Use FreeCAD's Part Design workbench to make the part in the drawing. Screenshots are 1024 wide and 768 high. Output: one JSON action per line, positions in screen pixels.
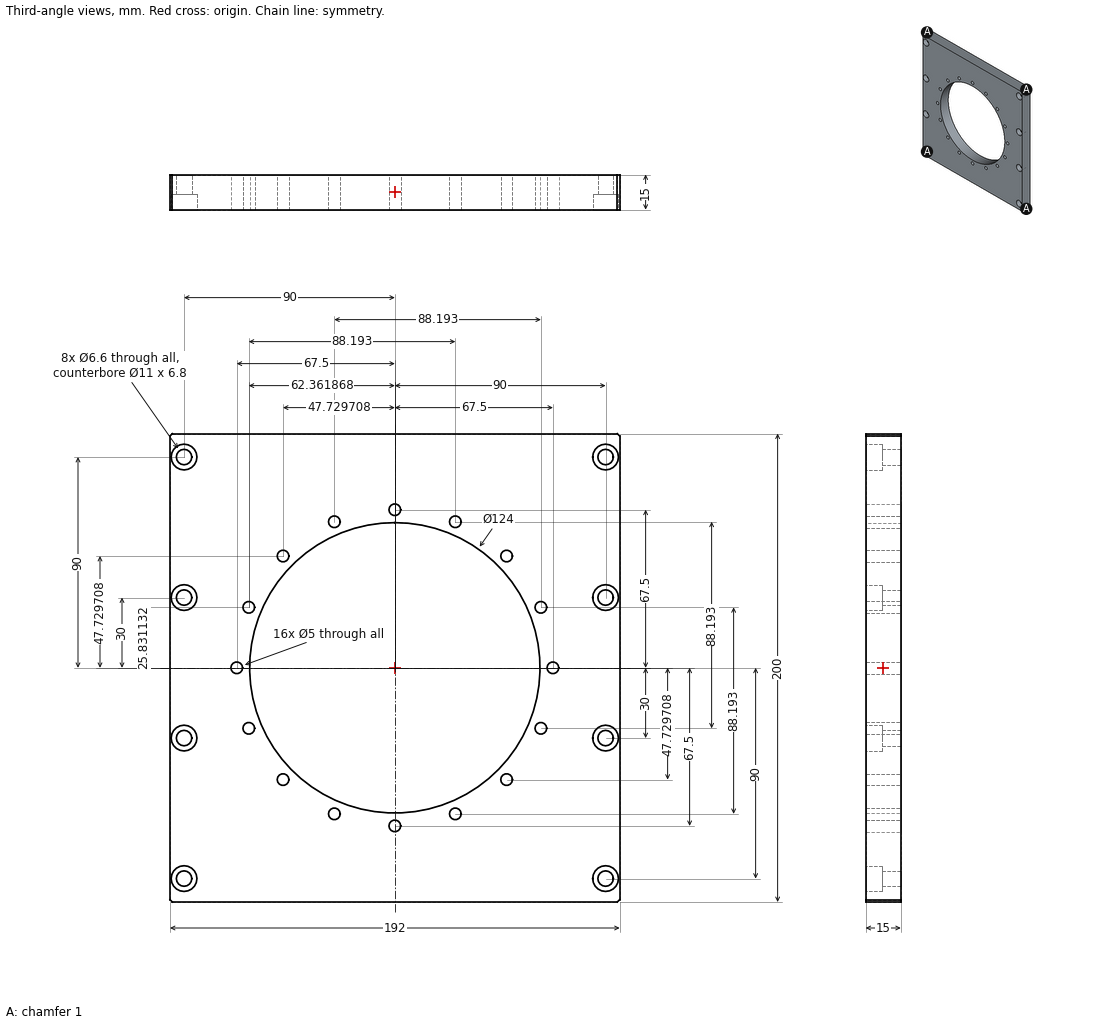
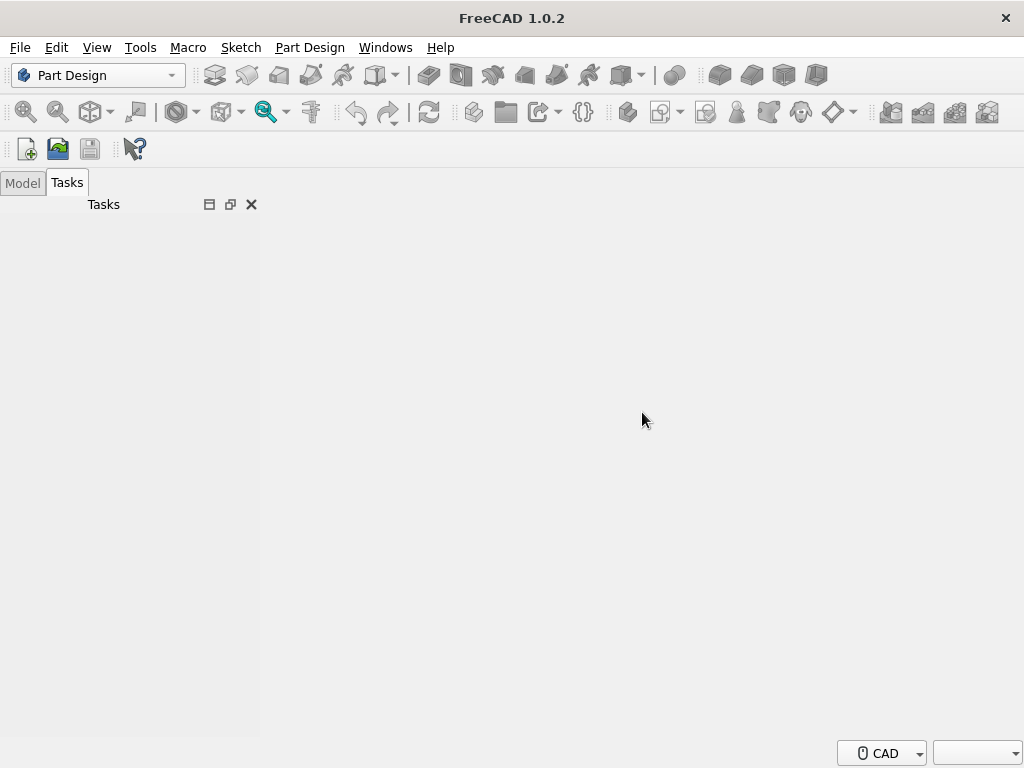
{"action": "left_click", "coordinate": [26, 150]}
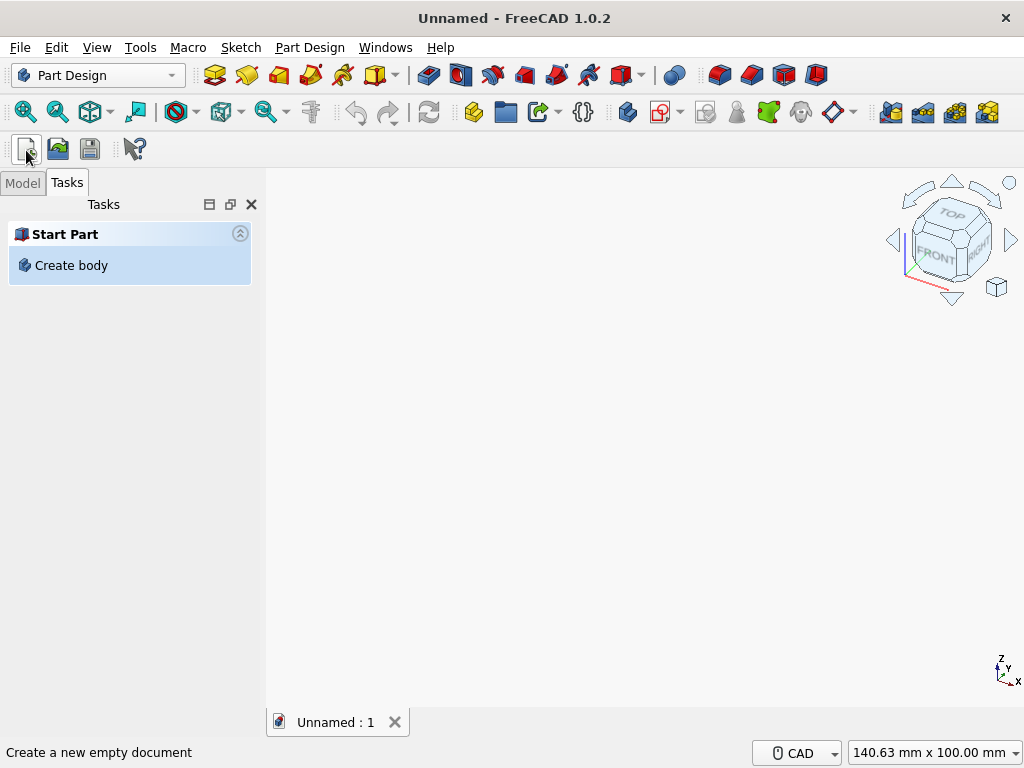
{"action": "left_click", "coordinate": [660, 112]}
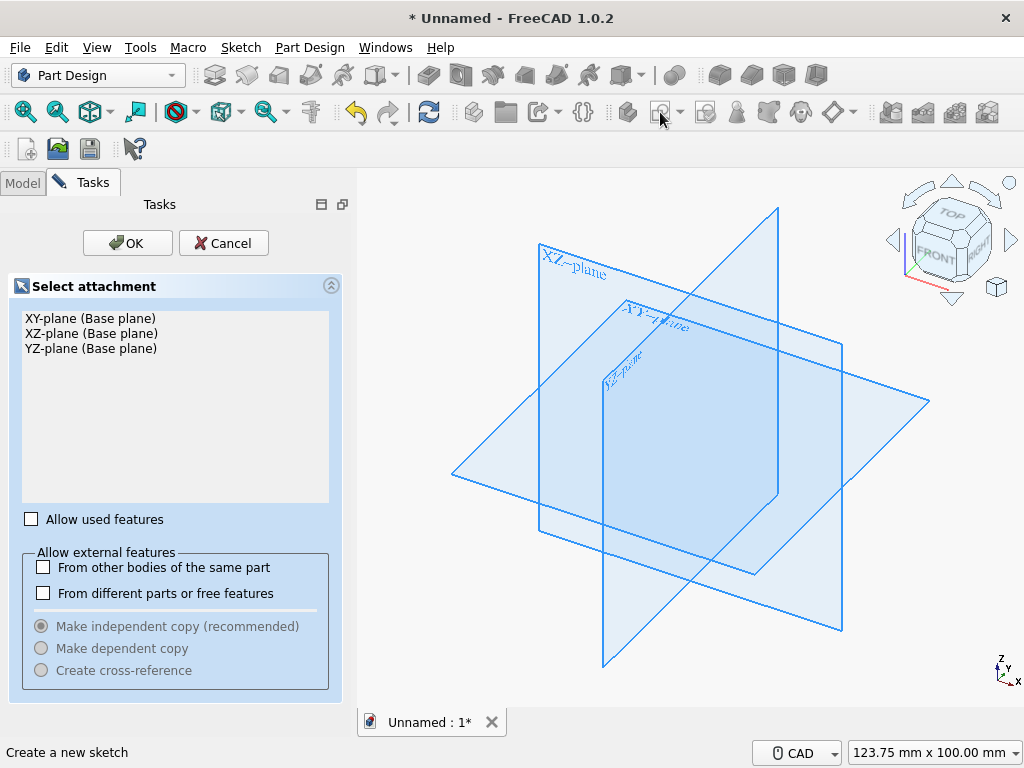
{"action": "left_click", "coordinate": [82, 334]}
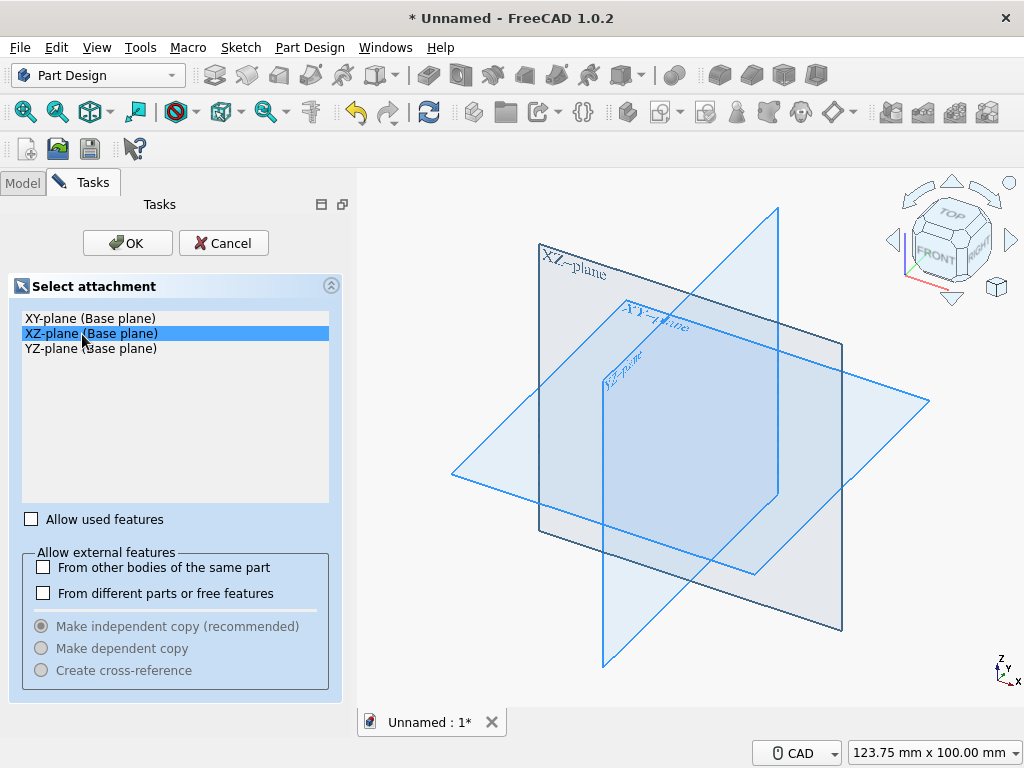
{"action": "left_click", "coordinate": [128, 243]}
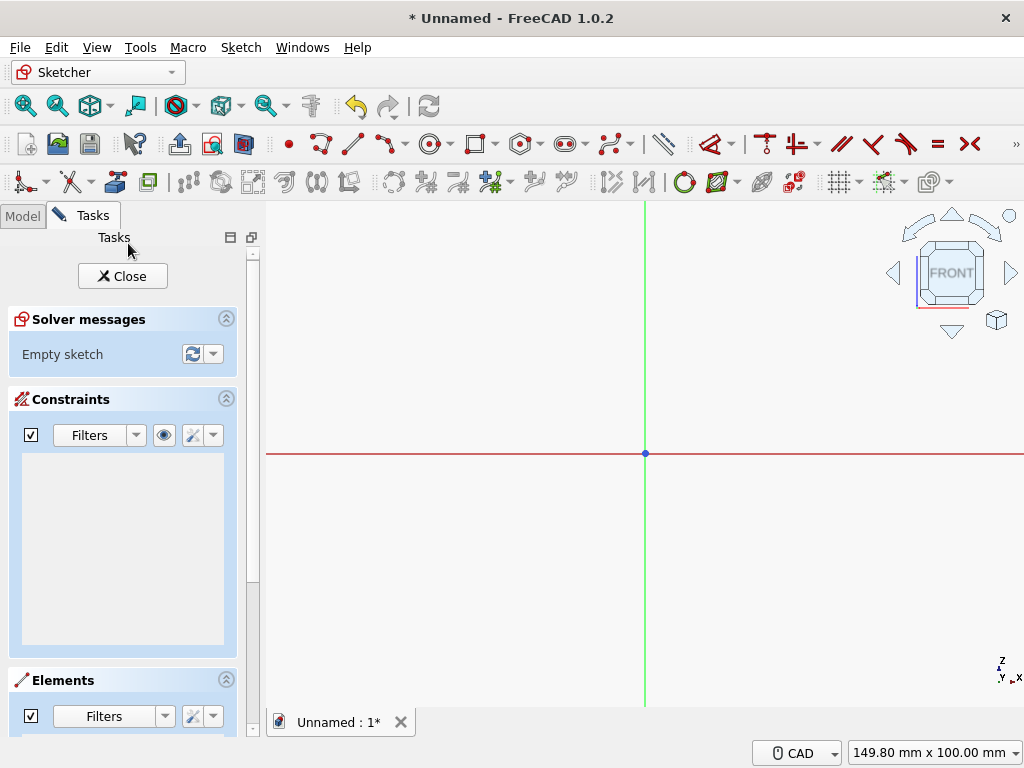
{"action": "scroll", "coordinate": [547, 454], "scroll_direction": "down", "scroll_amount": 6}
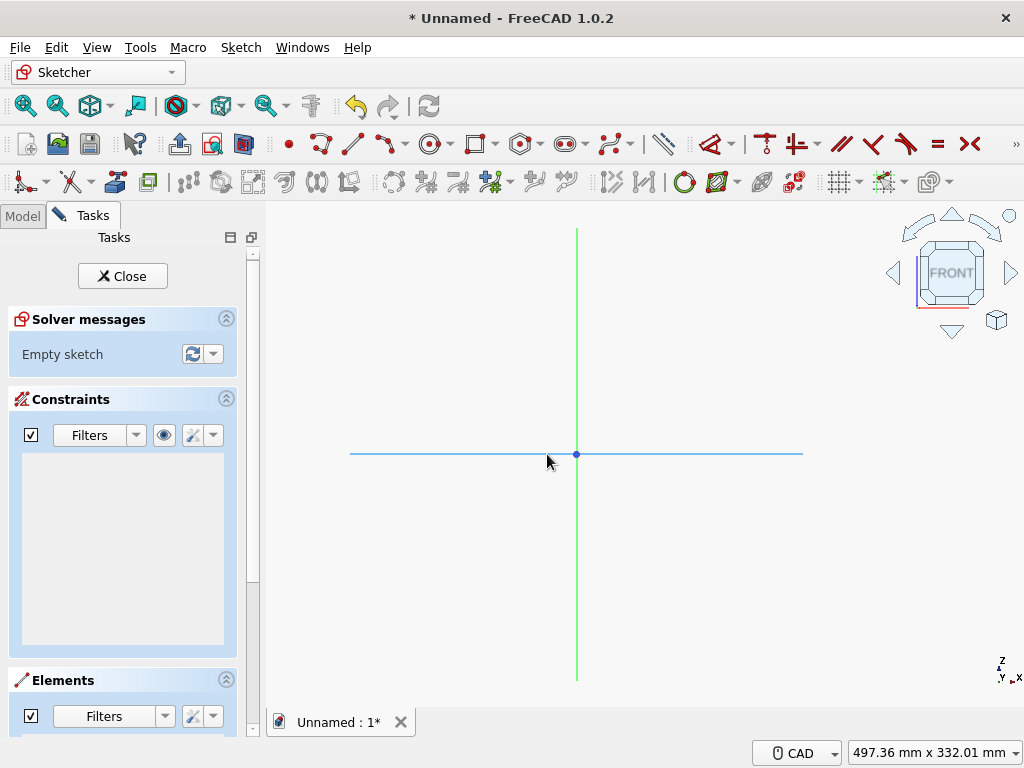
{"action": "left_click", "coordinate": [498, 144]}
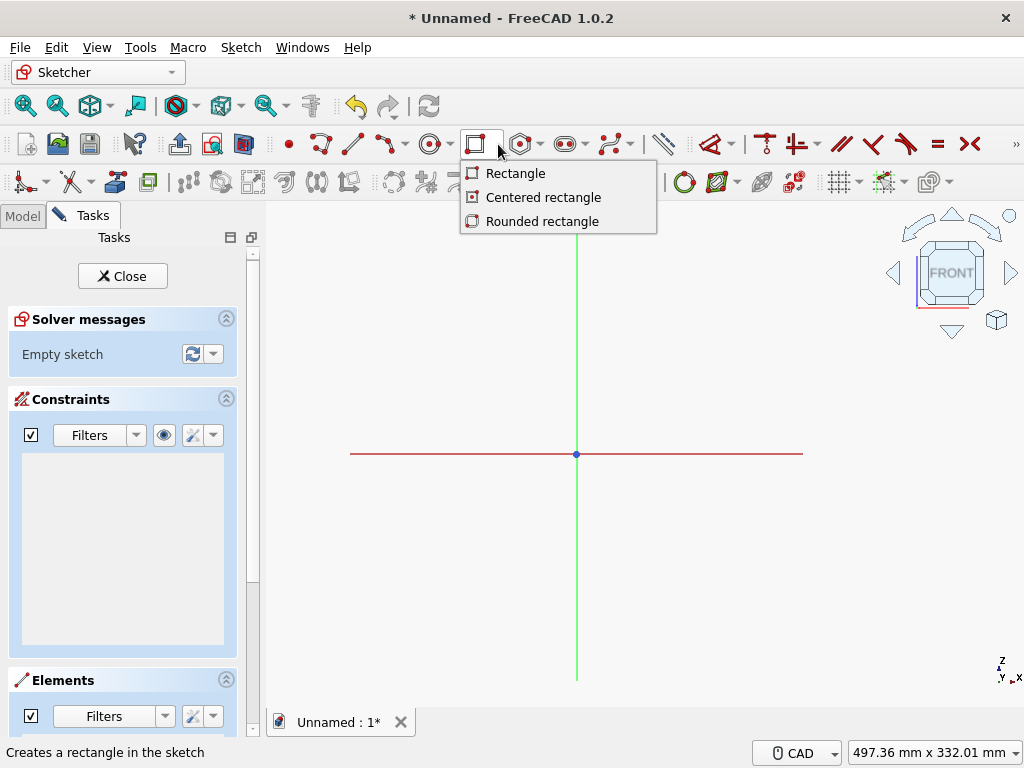
{"action": "left_click", "coordinate": [558, 197]}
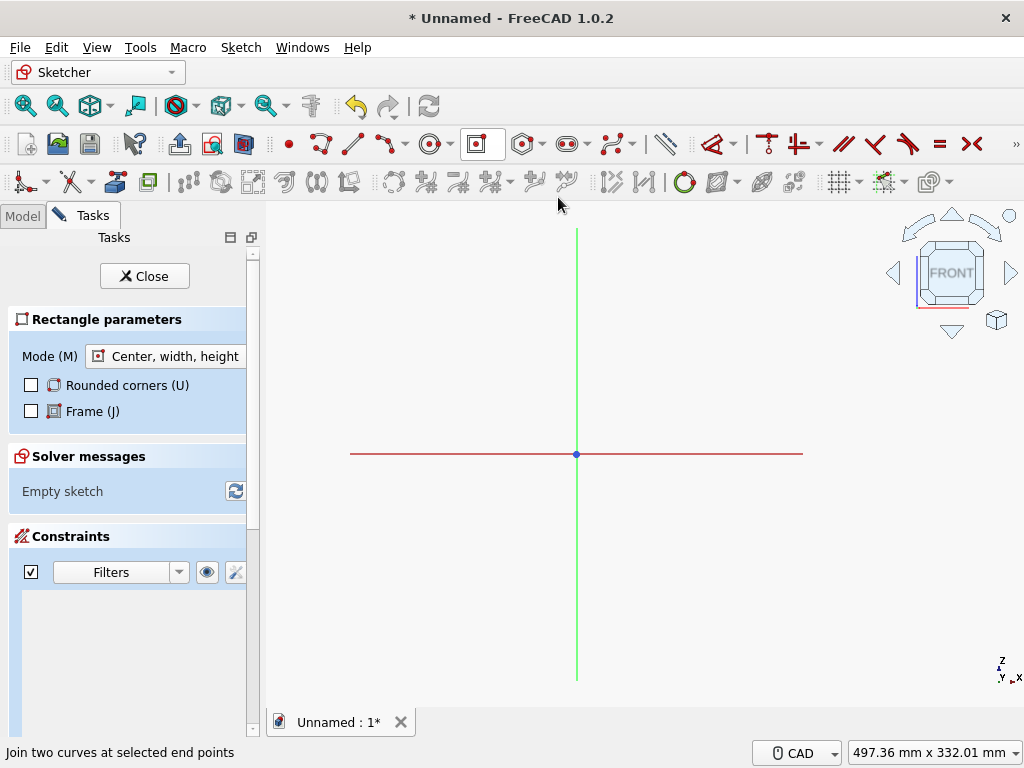
{"action": "left_click", "coordinate": [577, 454]}
{"action": "mouse_move", "coordinate": [723, 302]}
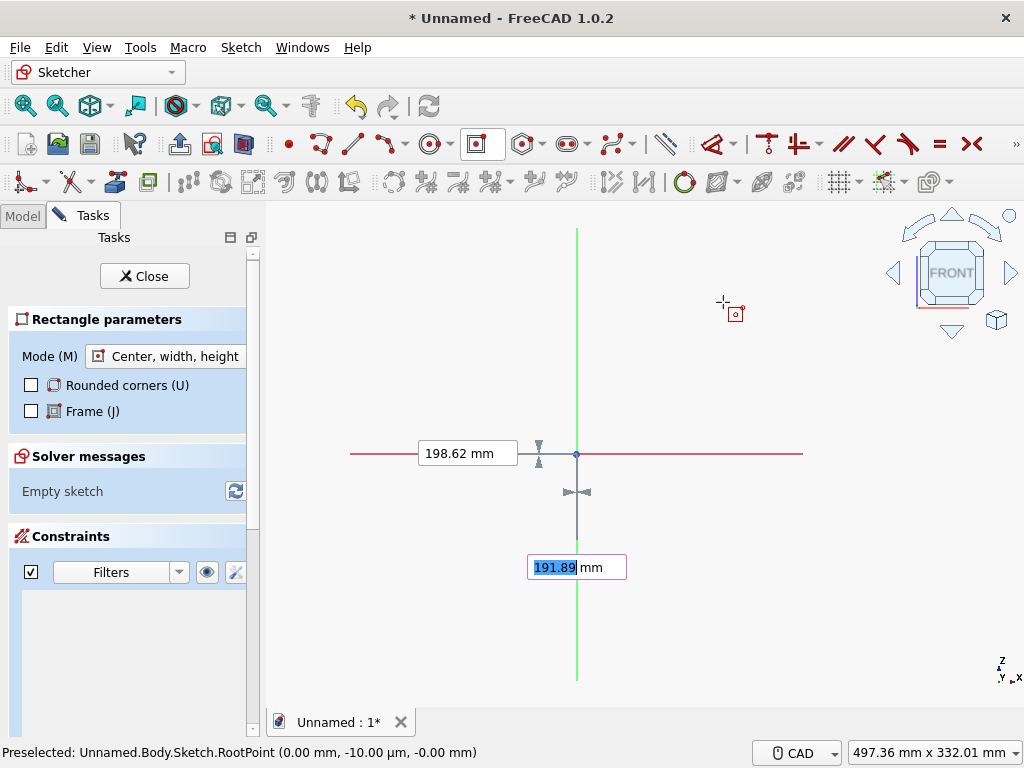
{"action": "type", "text": "192"}
{"action": "key", "text": "Tab"}
{"action": "type", "text": "200"}
{"action": "key", "text": "Return"}
{"action": "key", "text": "Escape"}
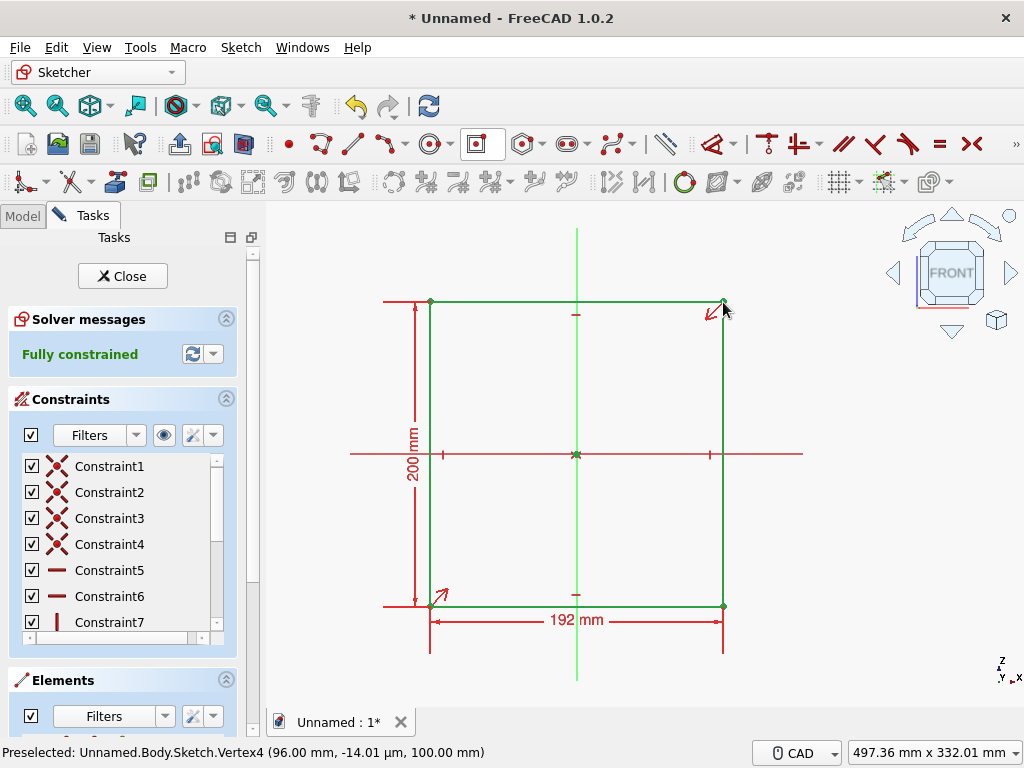
{"action": "left_click", "coordinate": [123, 276]}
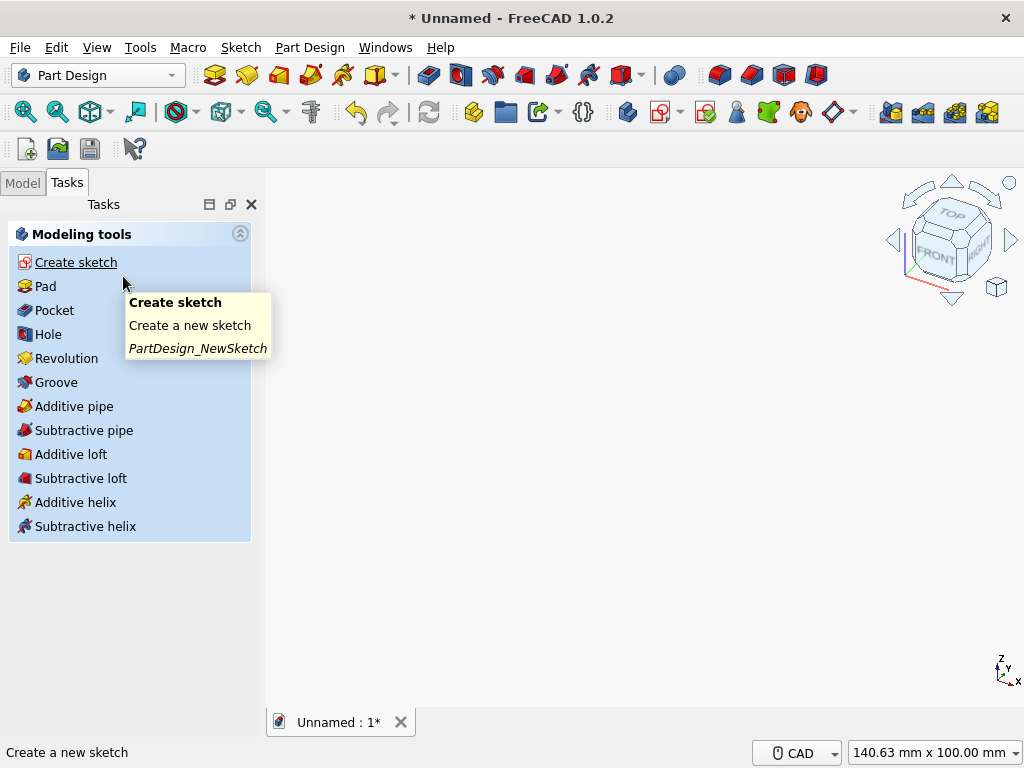
{"action": "left_click", "coordinate": [216, 76]}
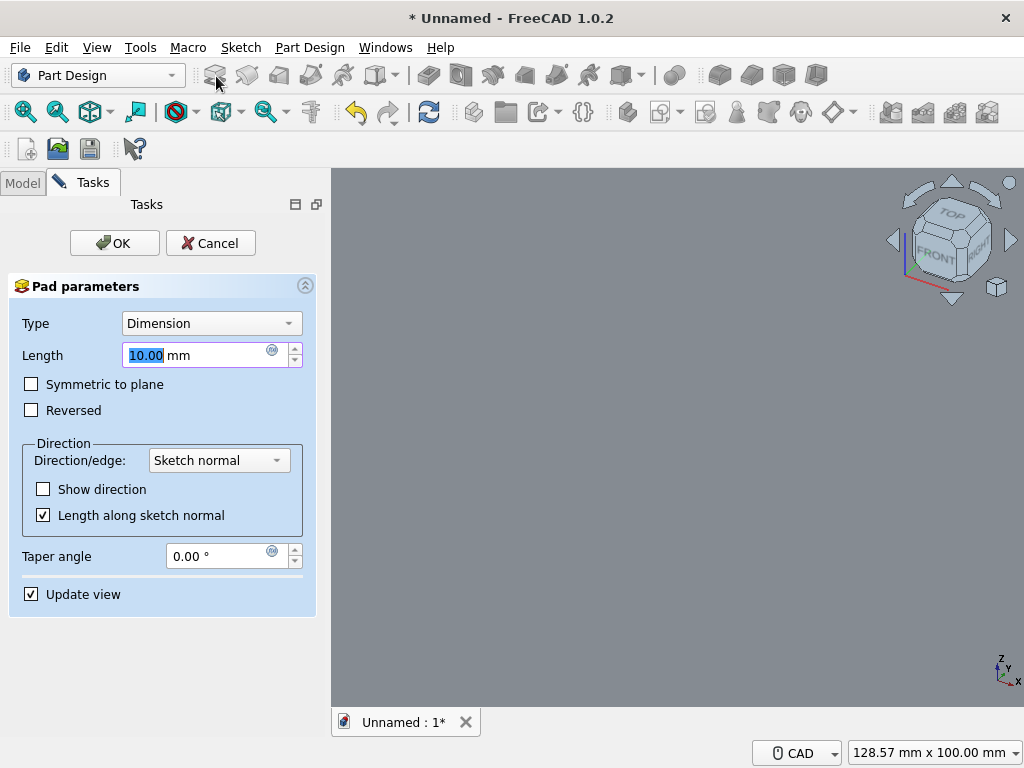
{"action": "type", "text": "15"}
{"action": "key", "text": "Tab"}